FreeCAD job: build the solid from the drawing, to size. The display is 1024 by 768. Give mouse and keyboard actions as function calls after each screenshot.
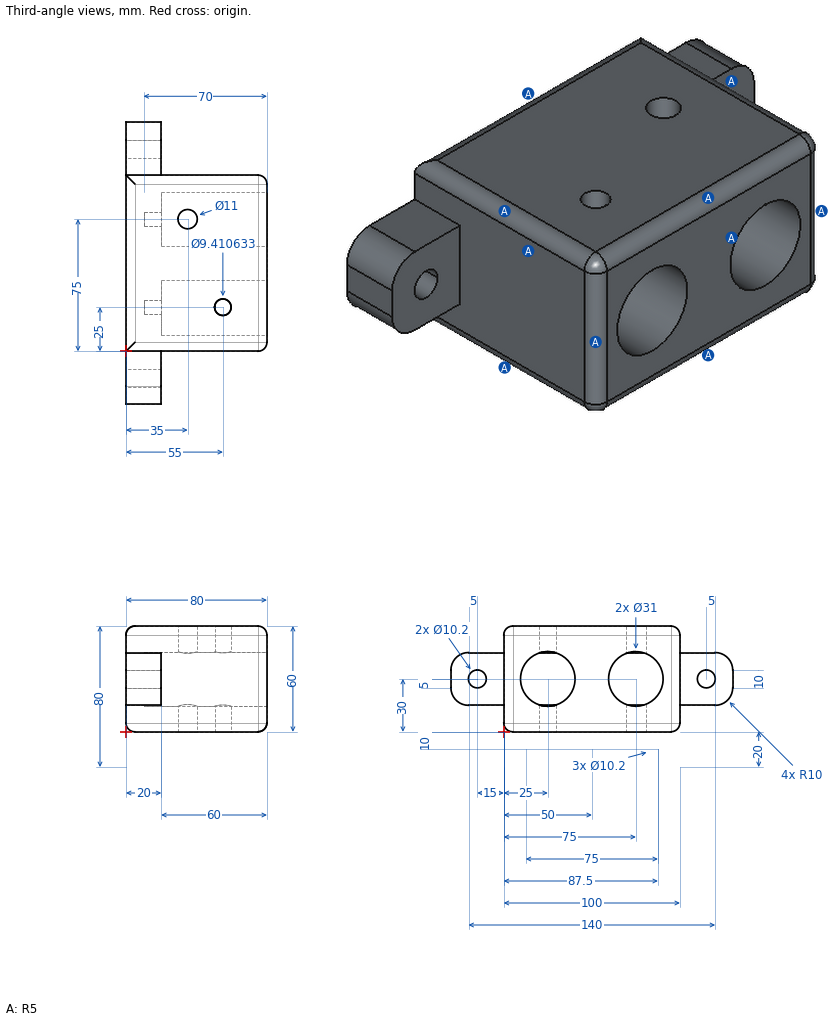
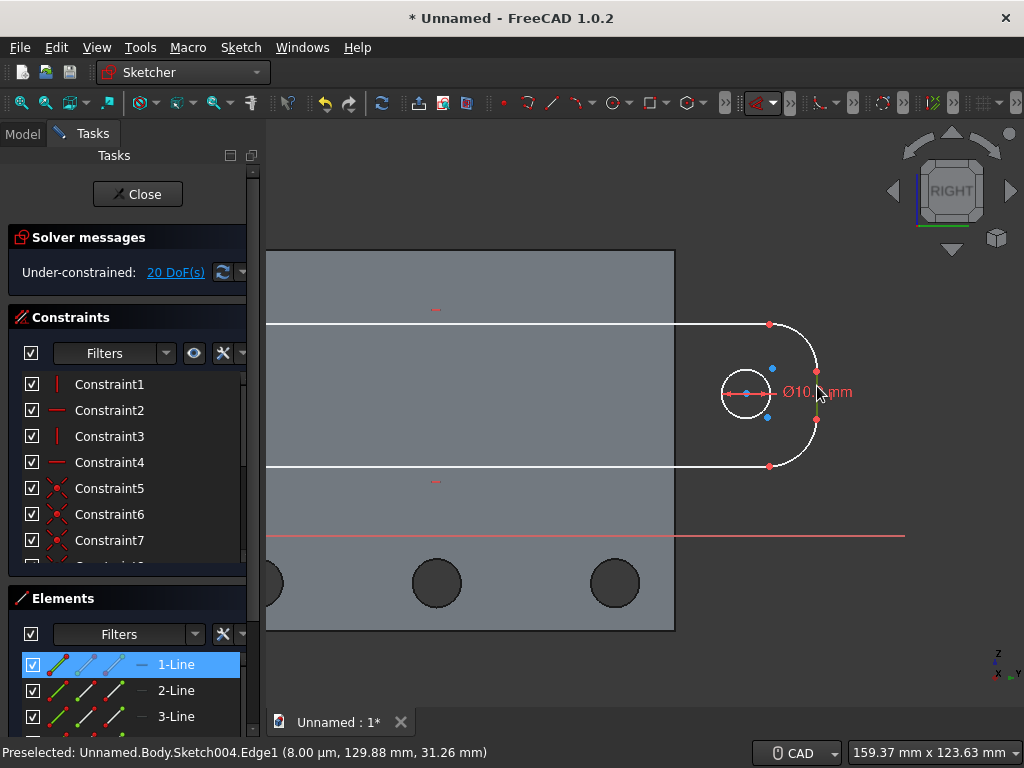
click(791, 461)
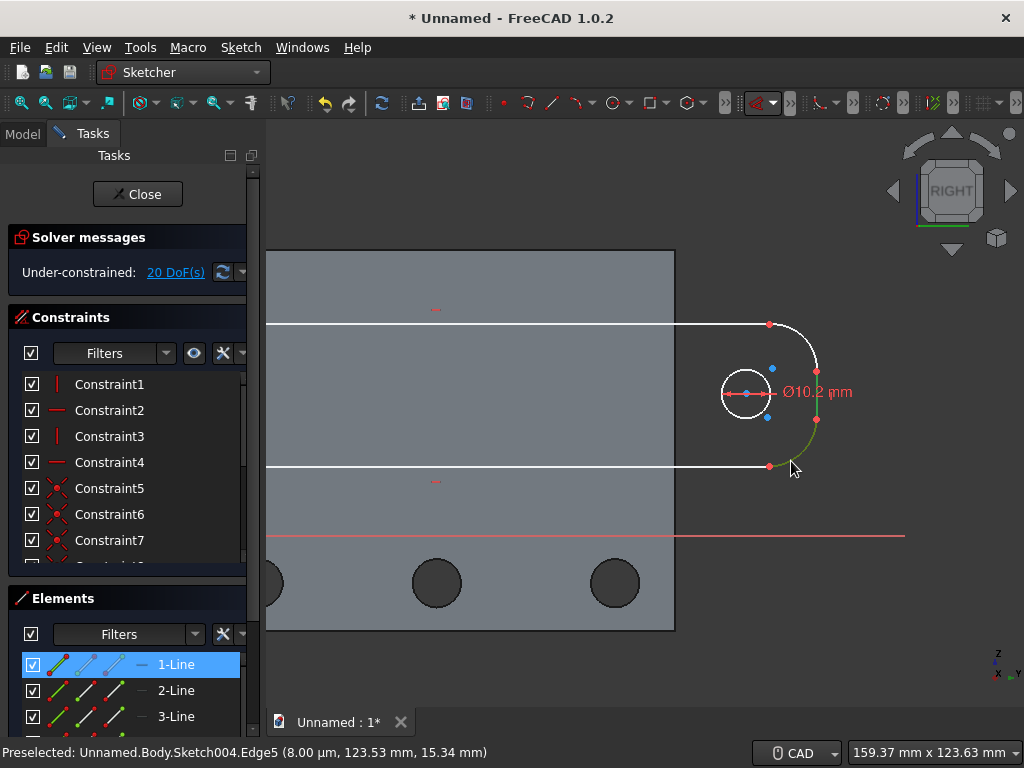
key(t)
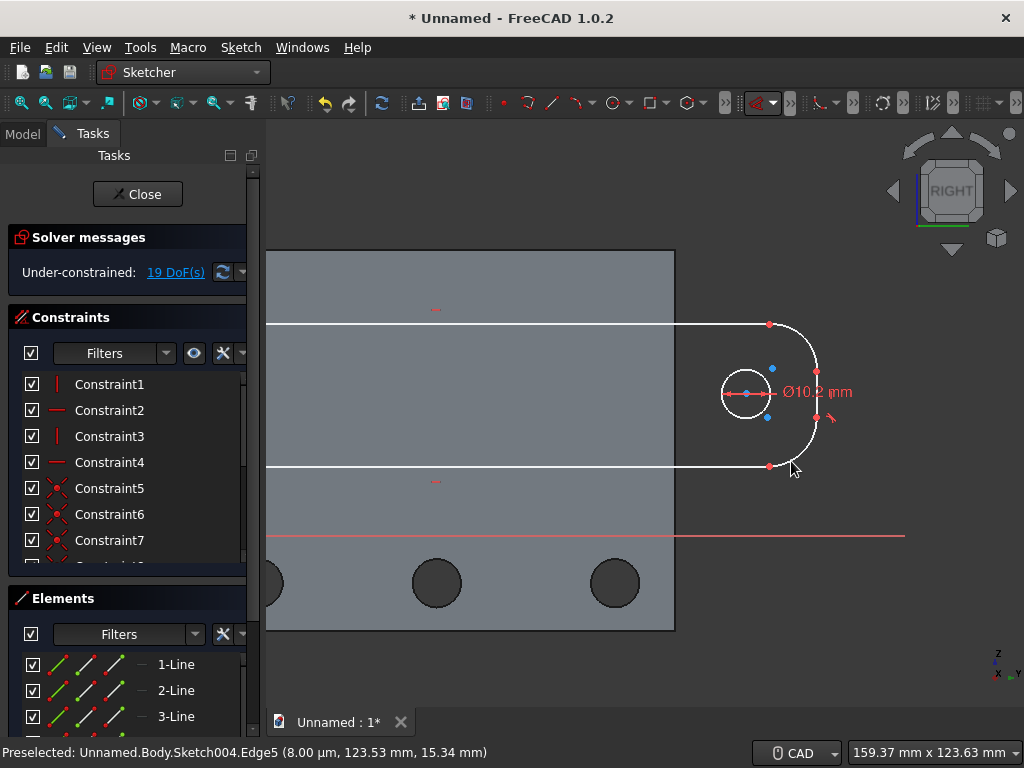
click(817, 385)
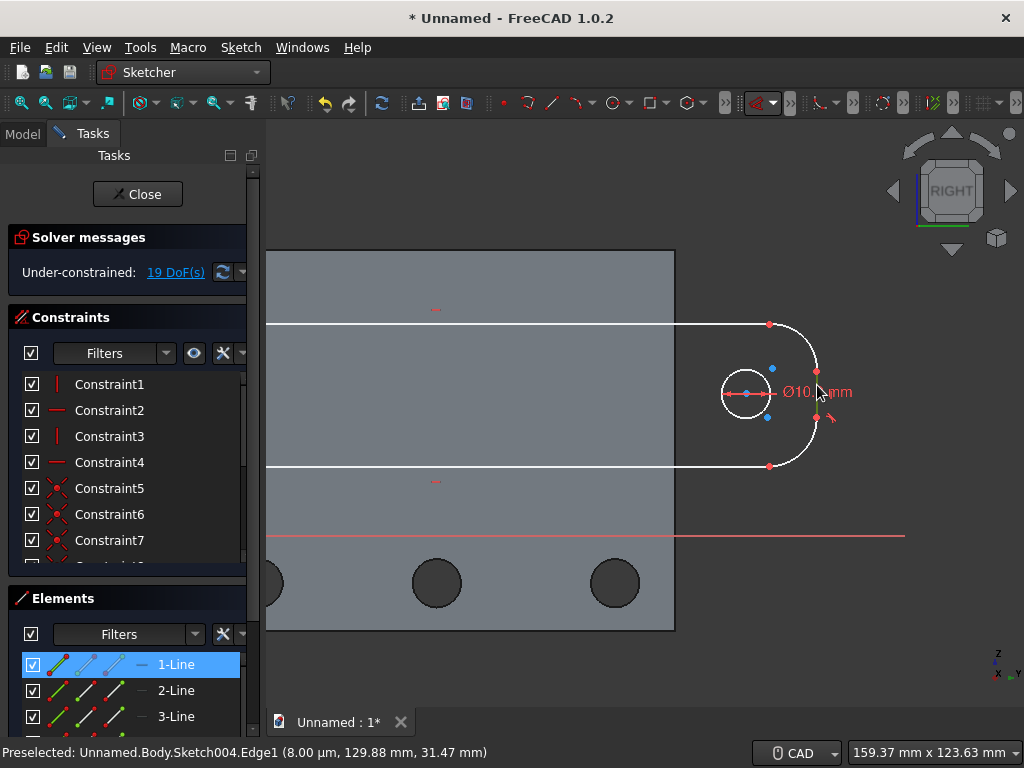
click(813, 350)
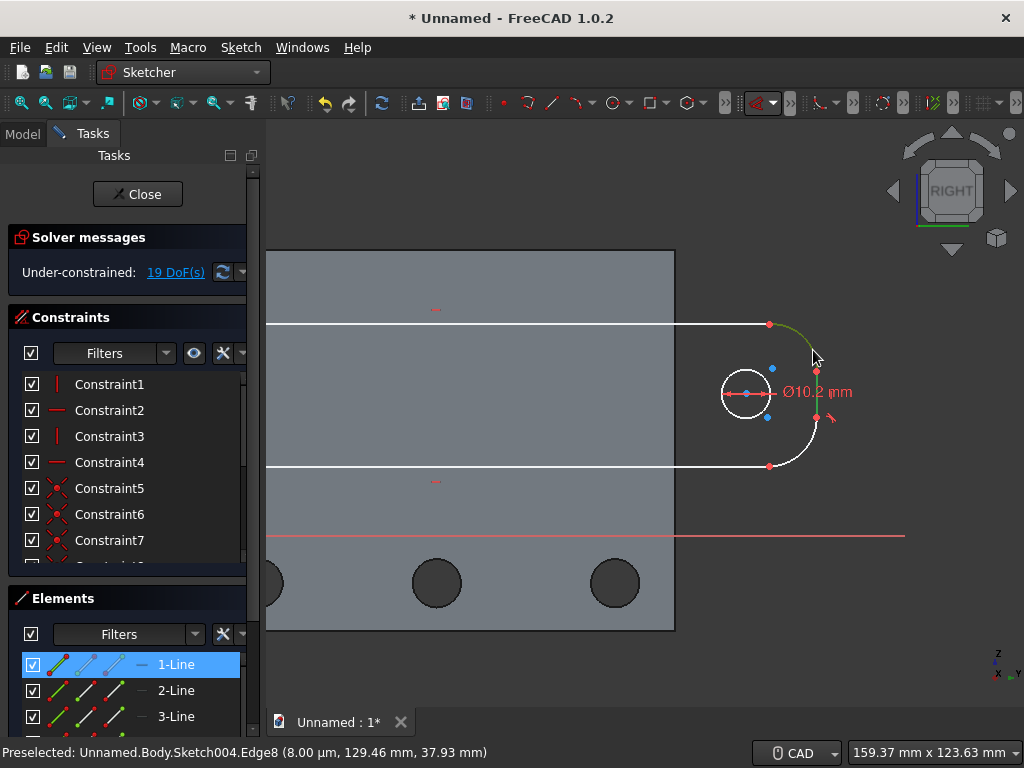
key(t)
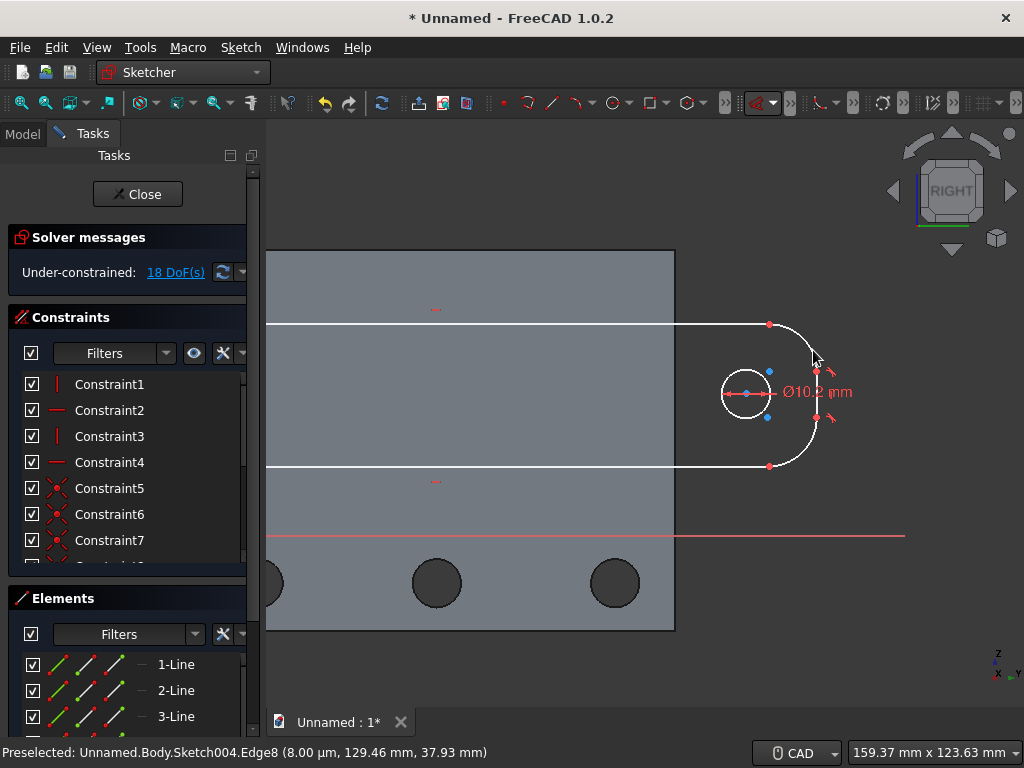
click(570, 467)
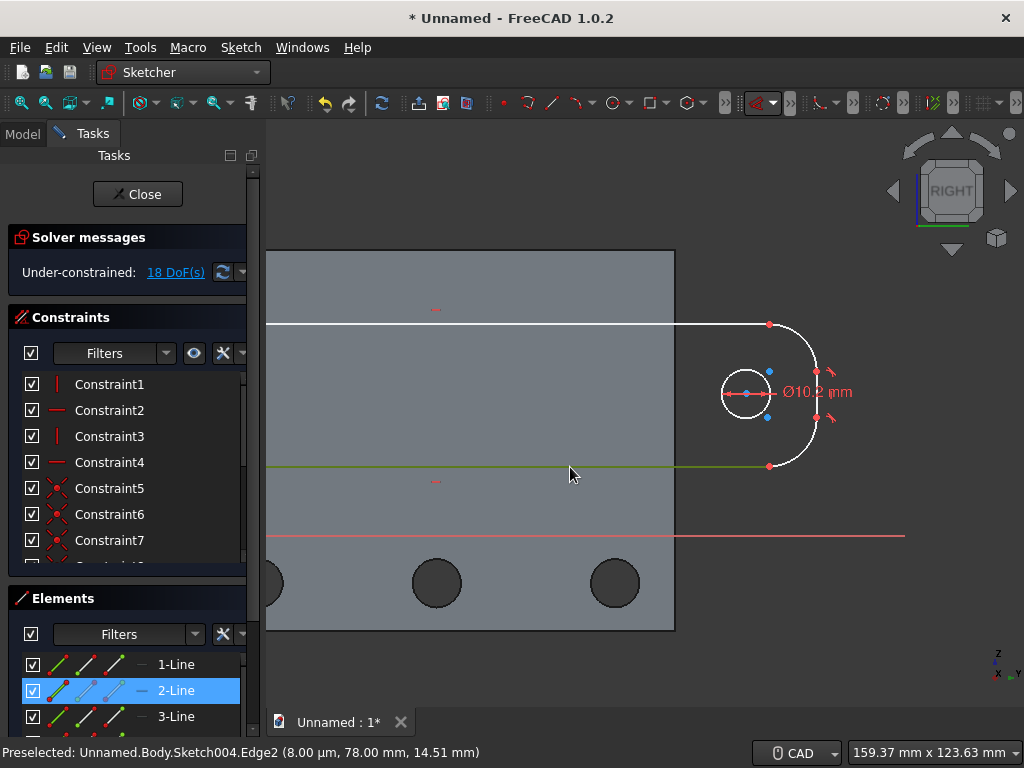
click(791, 461)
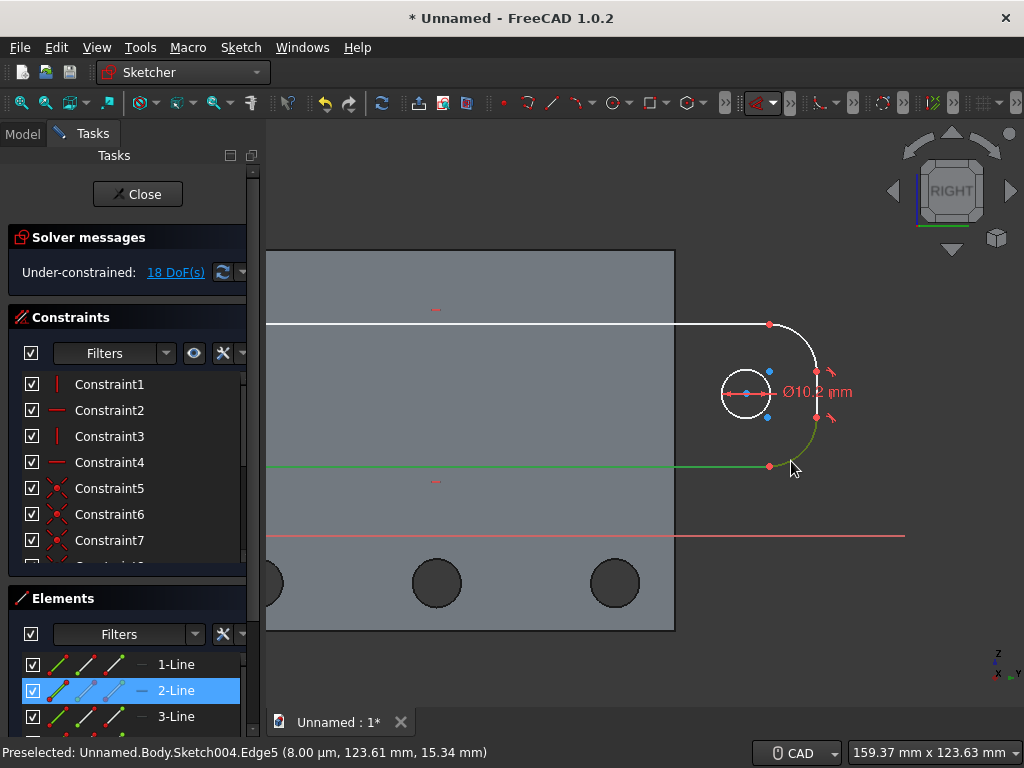
key(t)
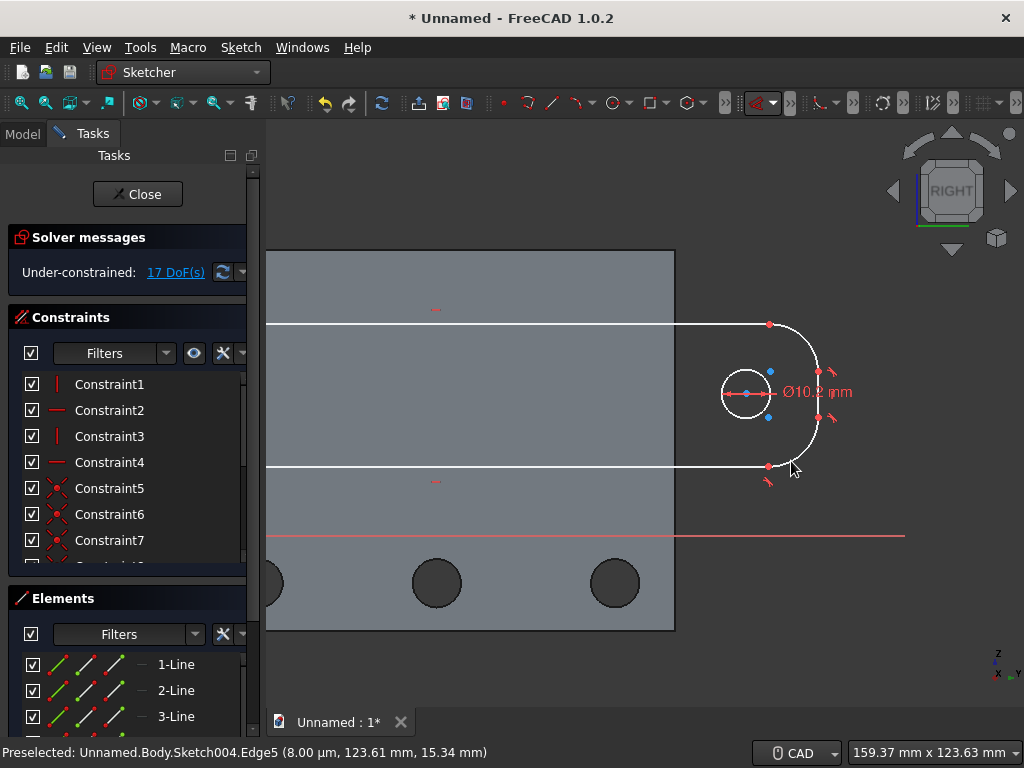
click(569, 467)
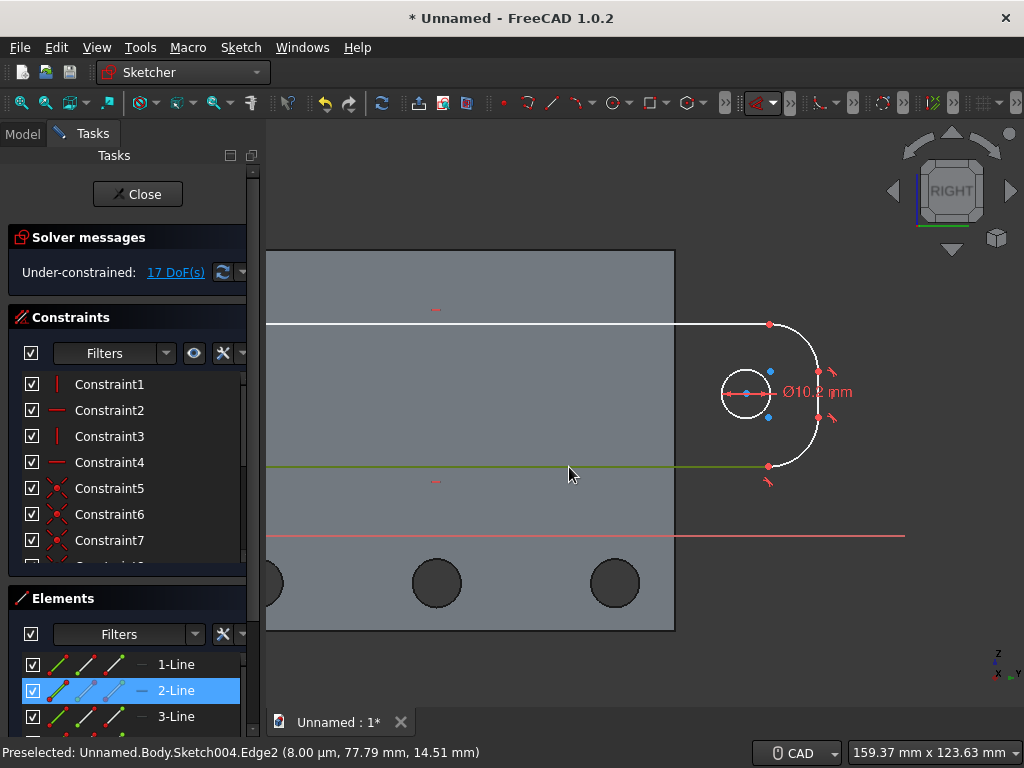
scroll(746, 394, down, 3)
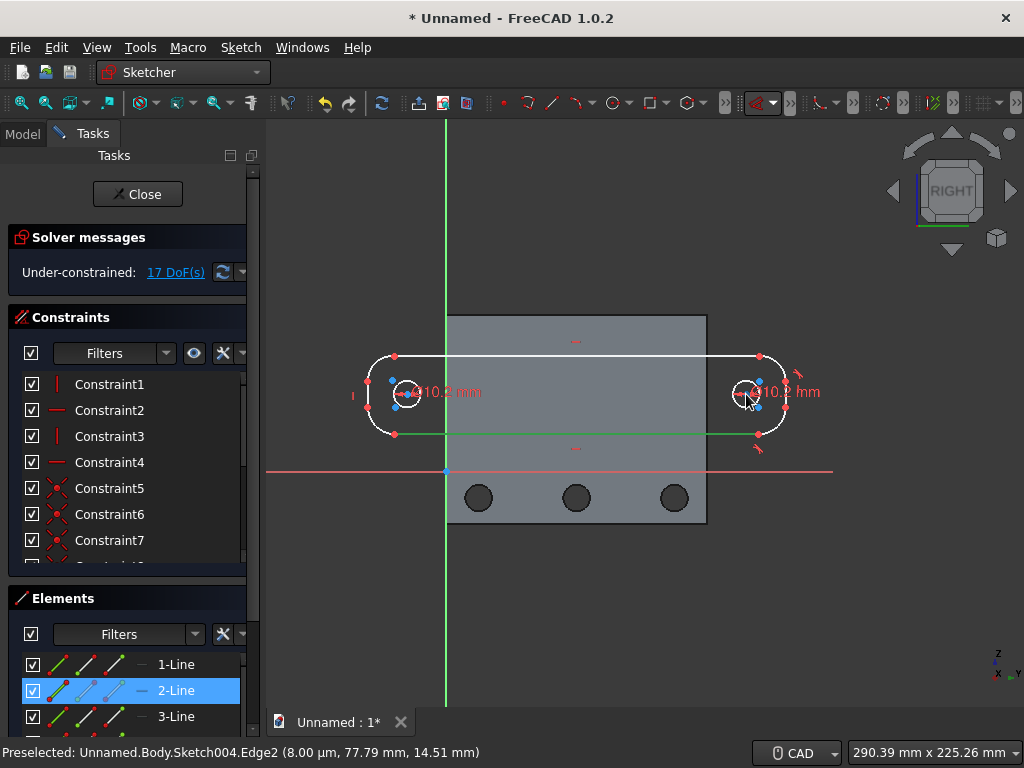
click(371, 420)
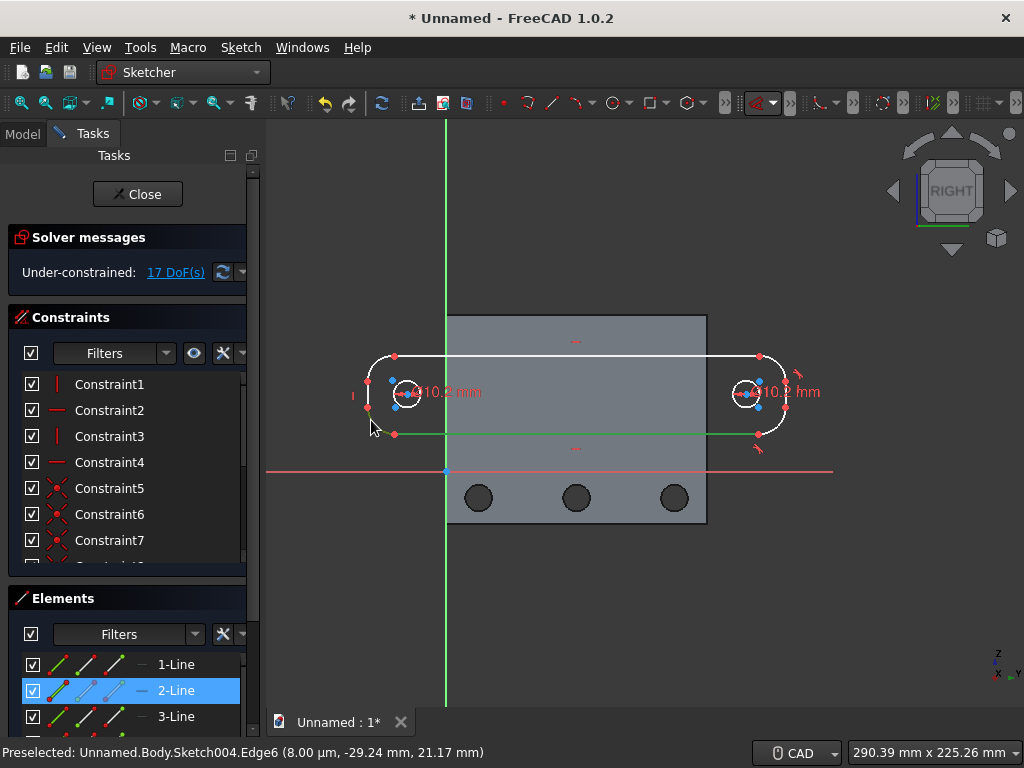
key(t)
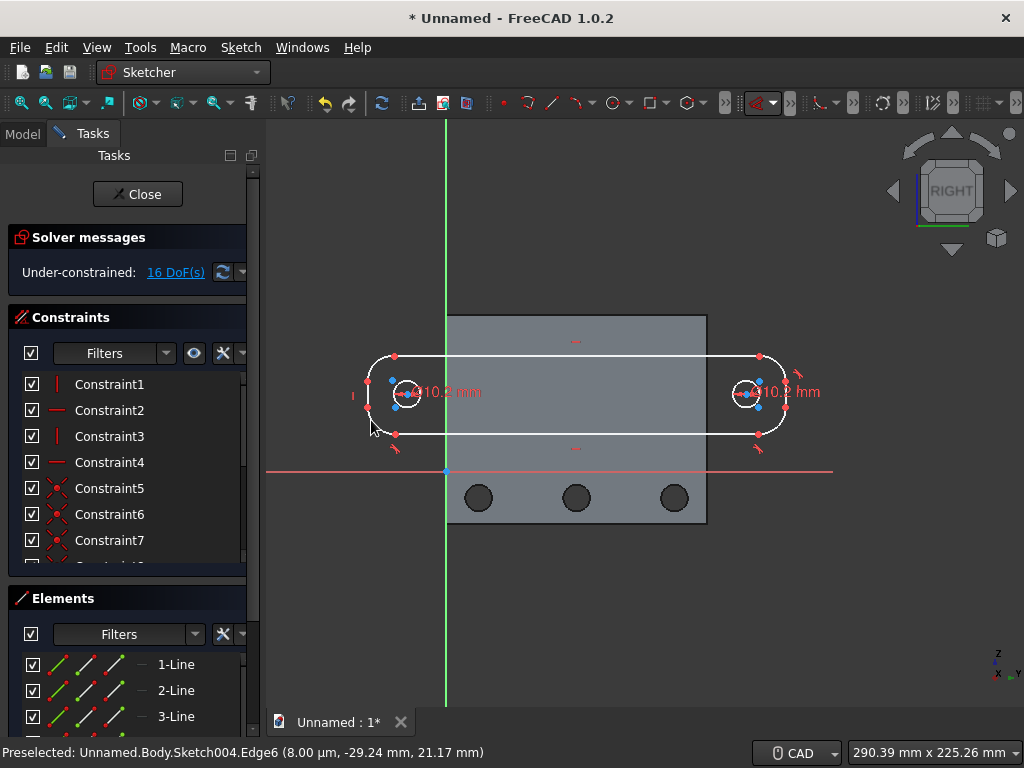
scroll(368, 398, up, 2)